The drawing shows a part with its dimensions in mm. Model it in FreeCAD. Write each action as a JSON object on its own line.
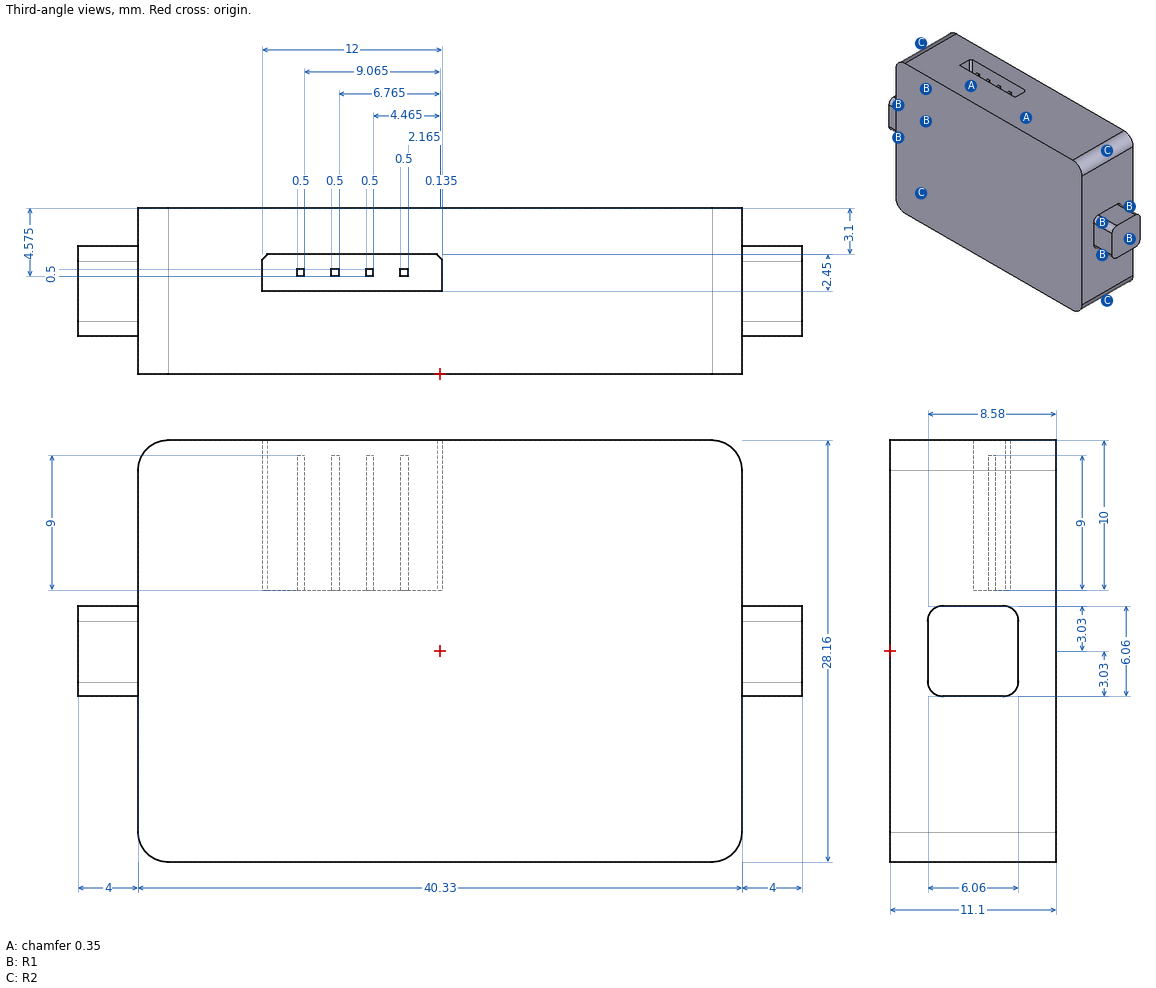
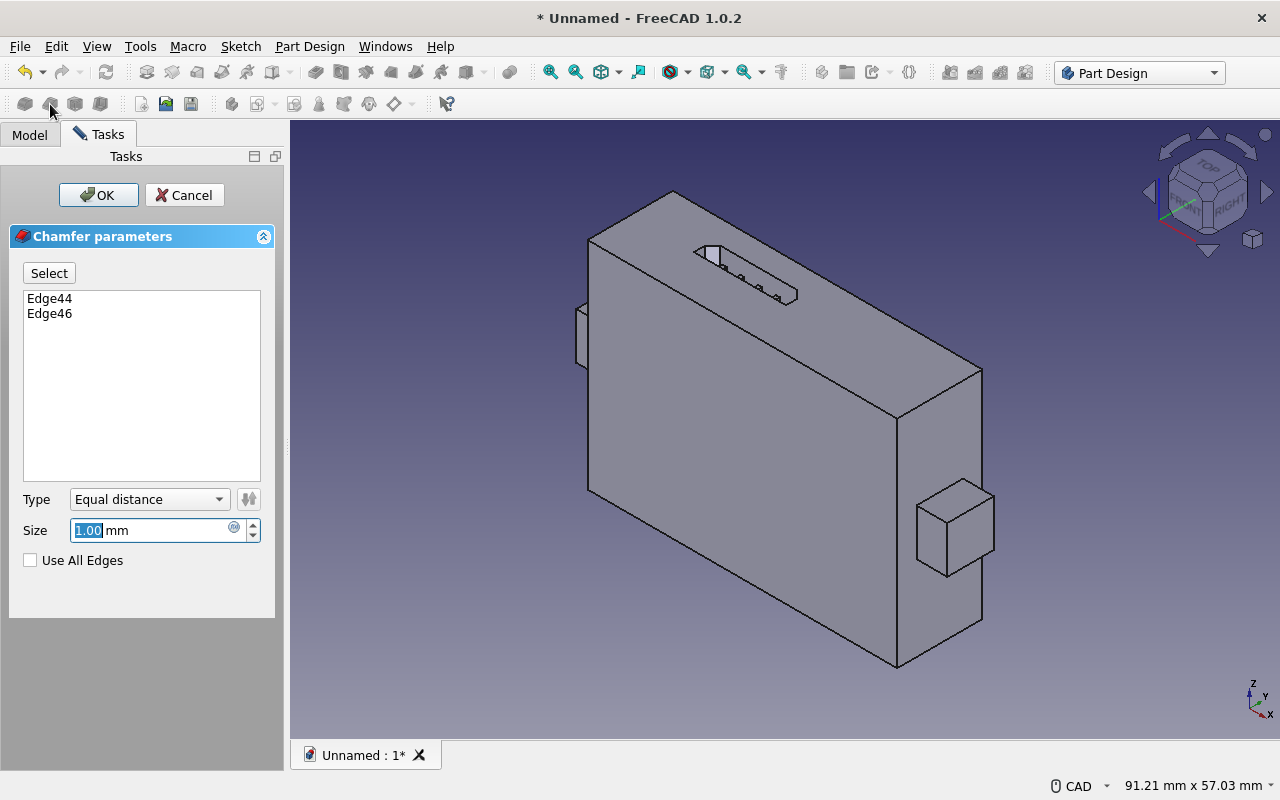
{"action": "type", "text": "0.35"}
{"action": "key", "text": "Tab"}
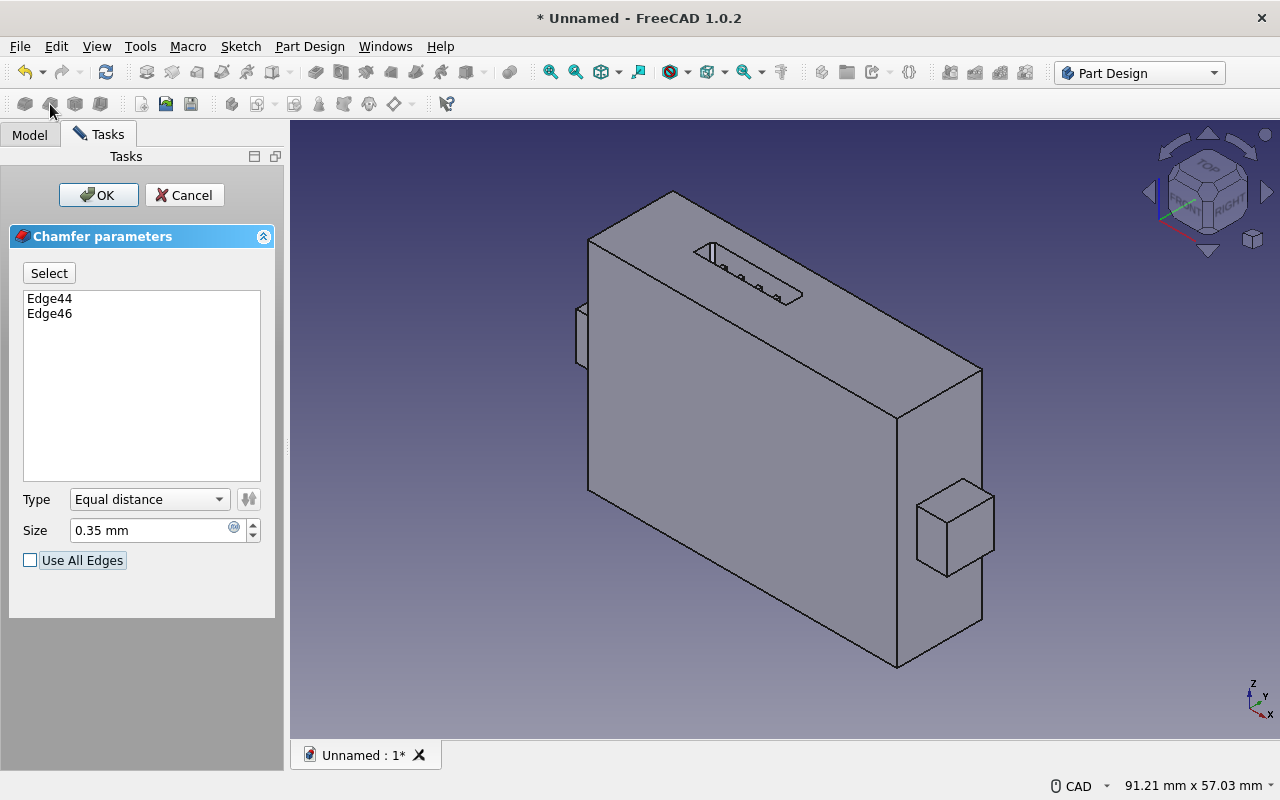
{"action": "left_click", "coordinate": [99, 195]}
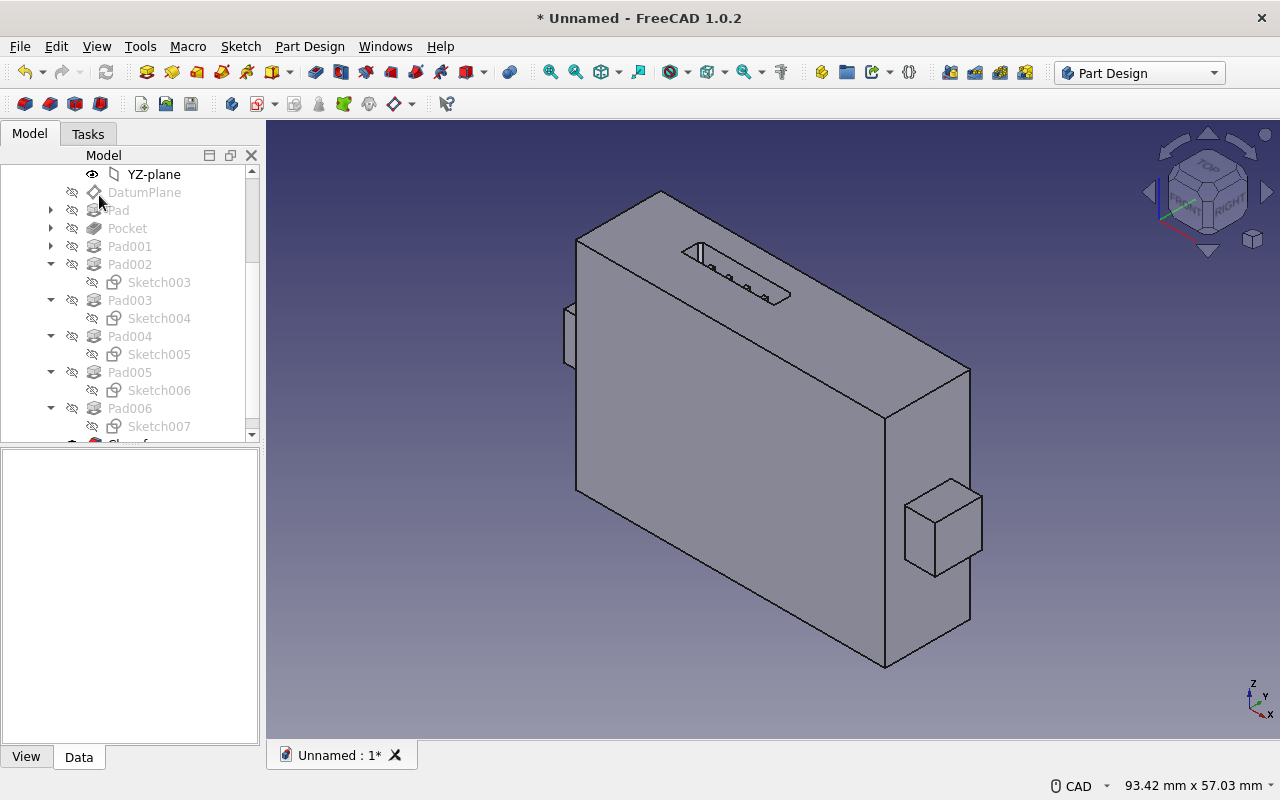
{"action": "left_click", "coordinate": [568, 310]}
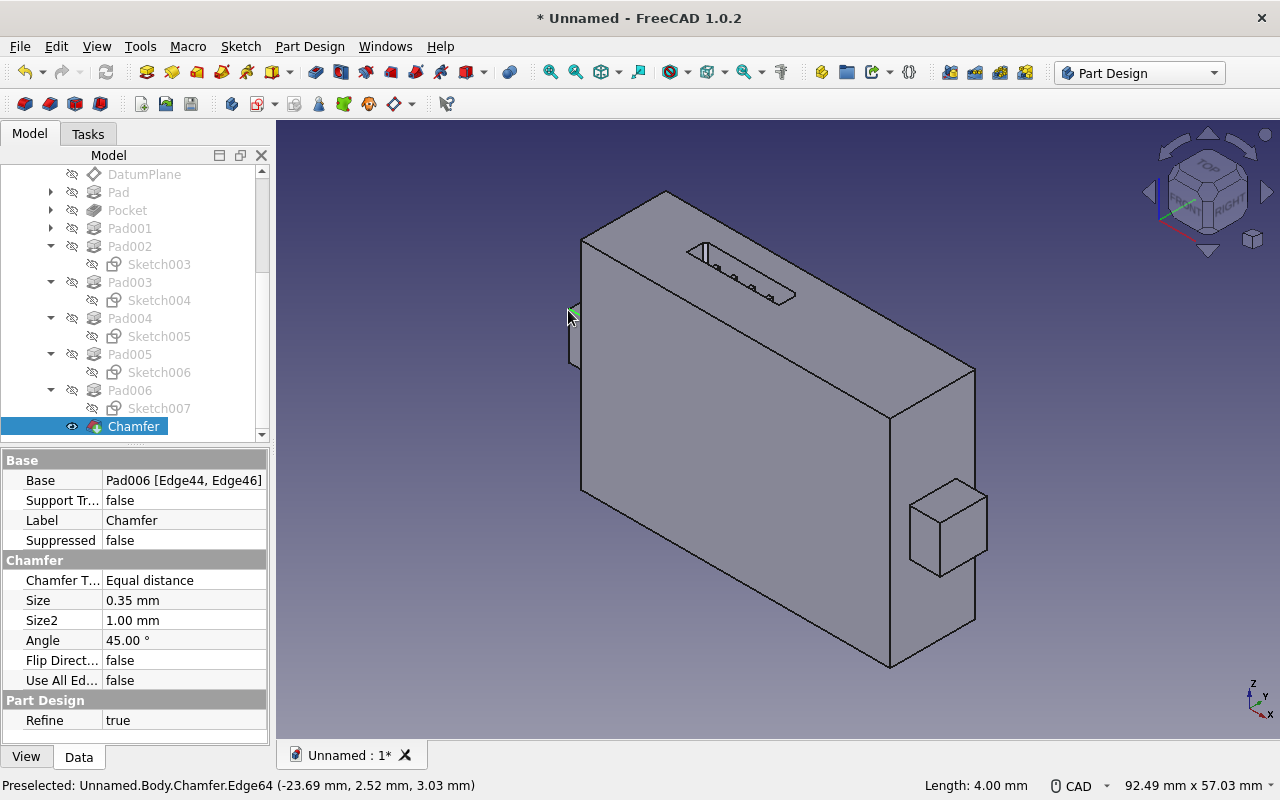
{"action": "left_click", "coordinate": [925, 513], "text": "ctrl"}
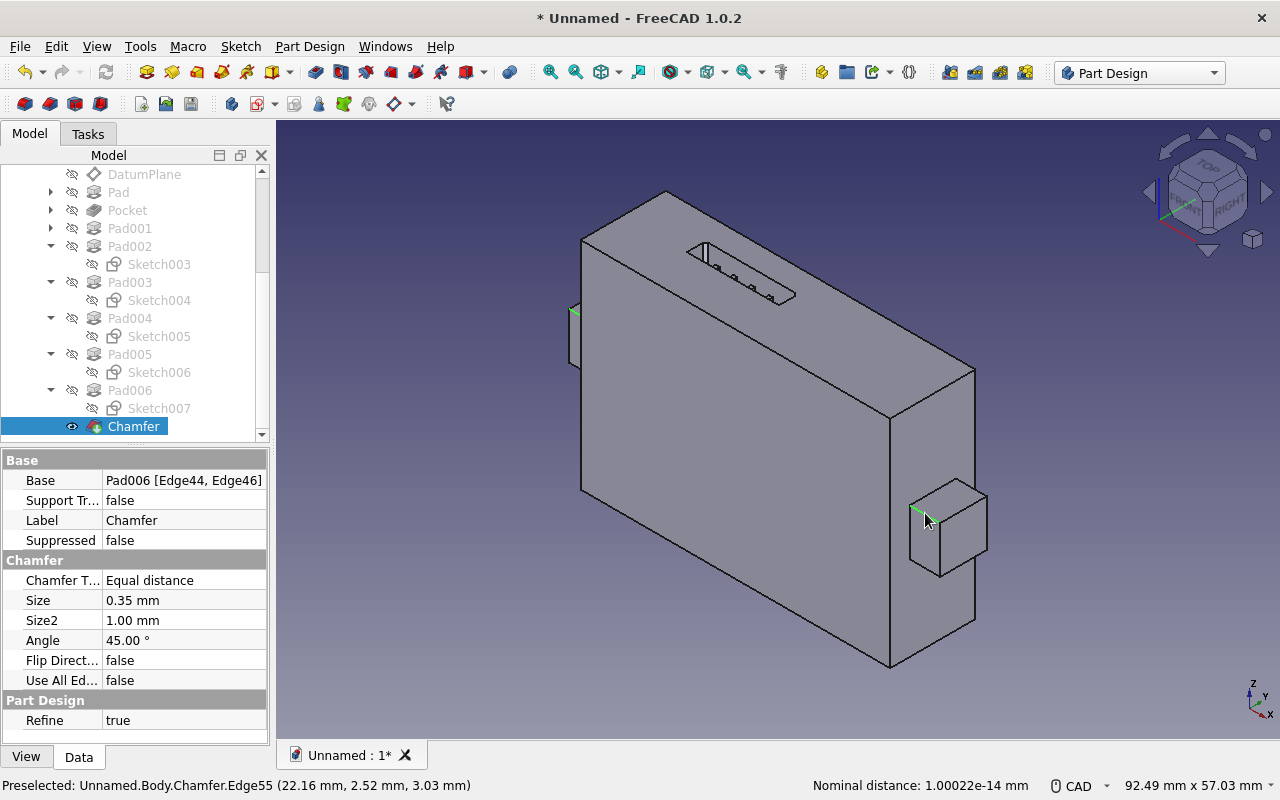
{"action": "key", "text": "2"}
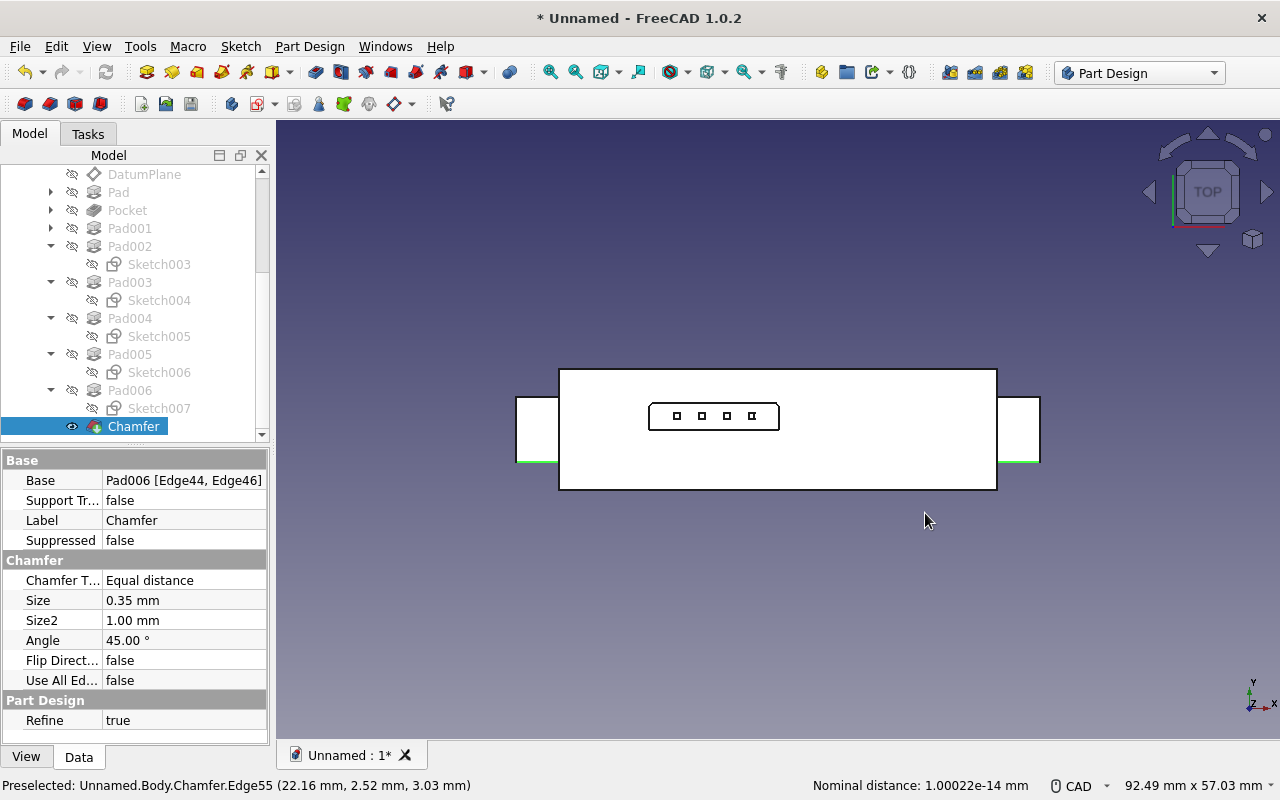
{"action": "left_click", "coordinate": [537, 396], "text": "ctrl"}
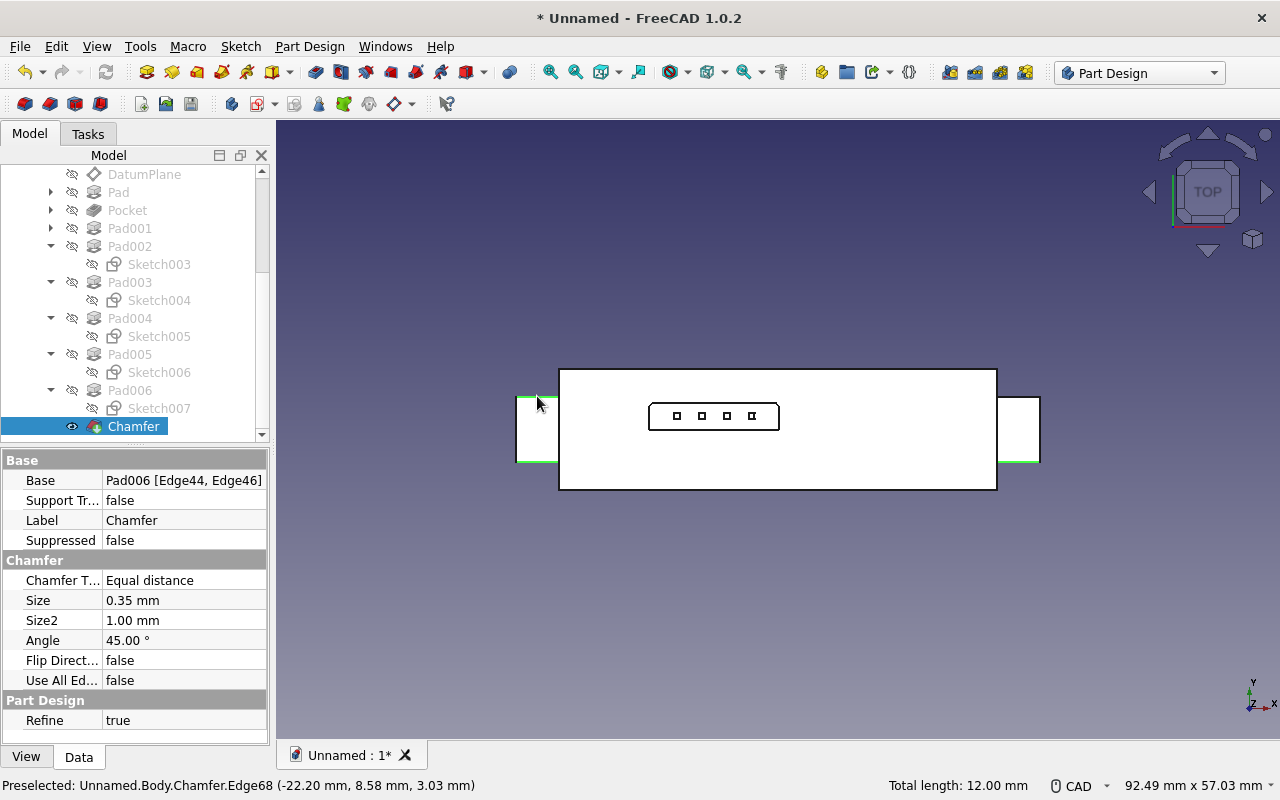
{"action": "left_click", "coordinate": [1019, 396], "text": "ctrl"}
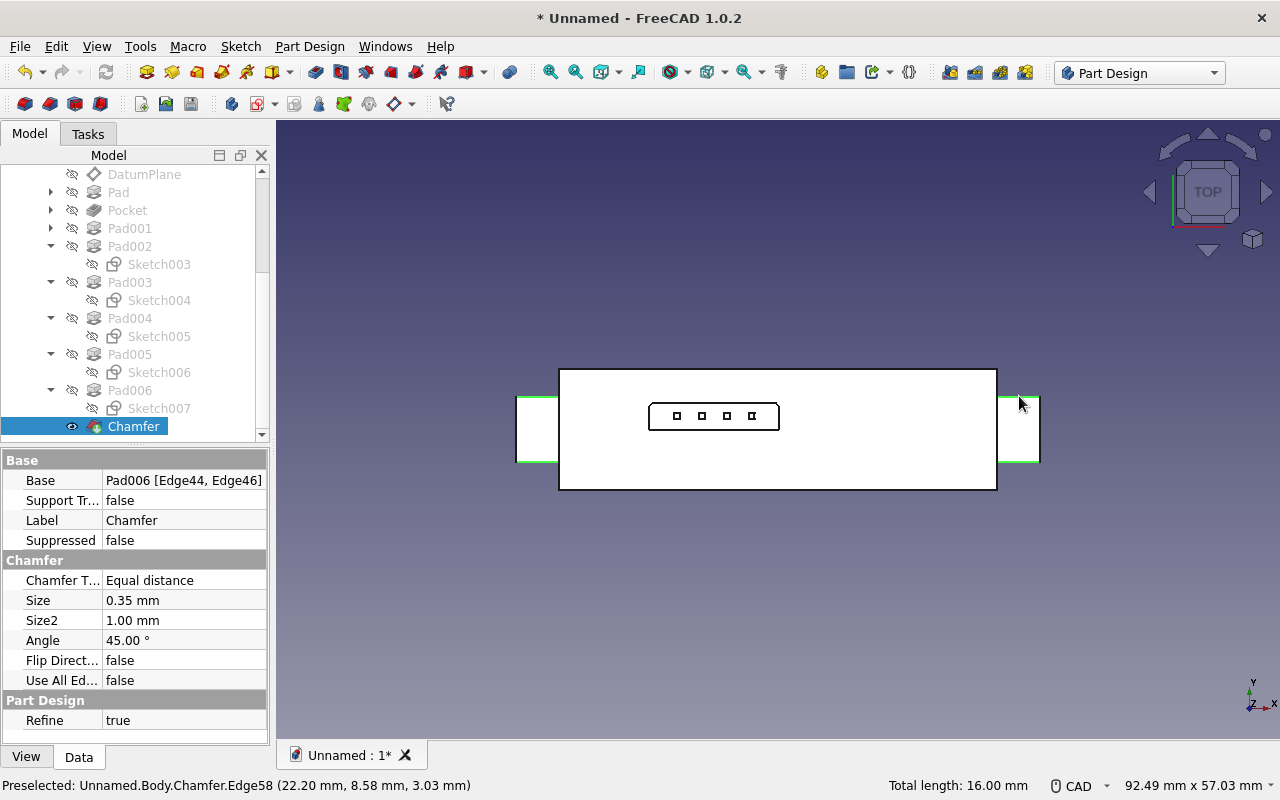
{"action": "key", "text": "0"}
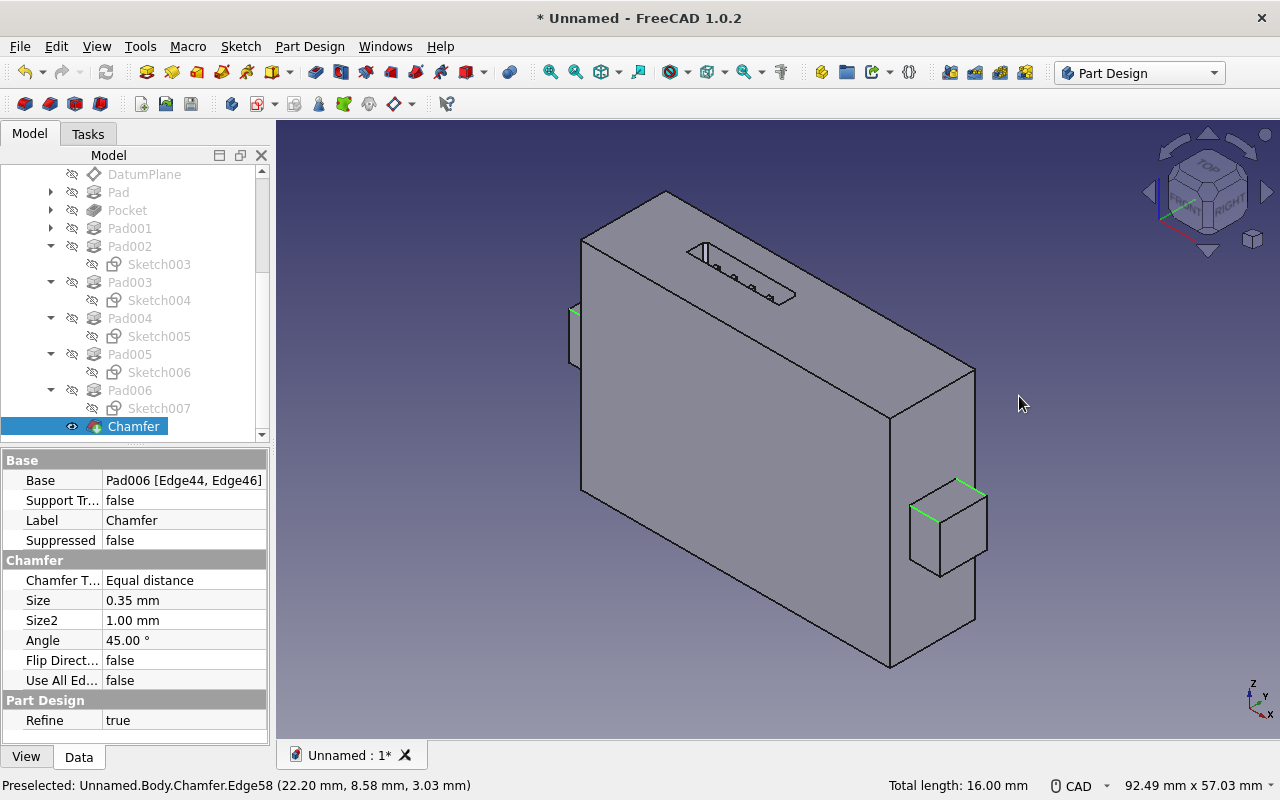
{"action": "key", "text": "1"}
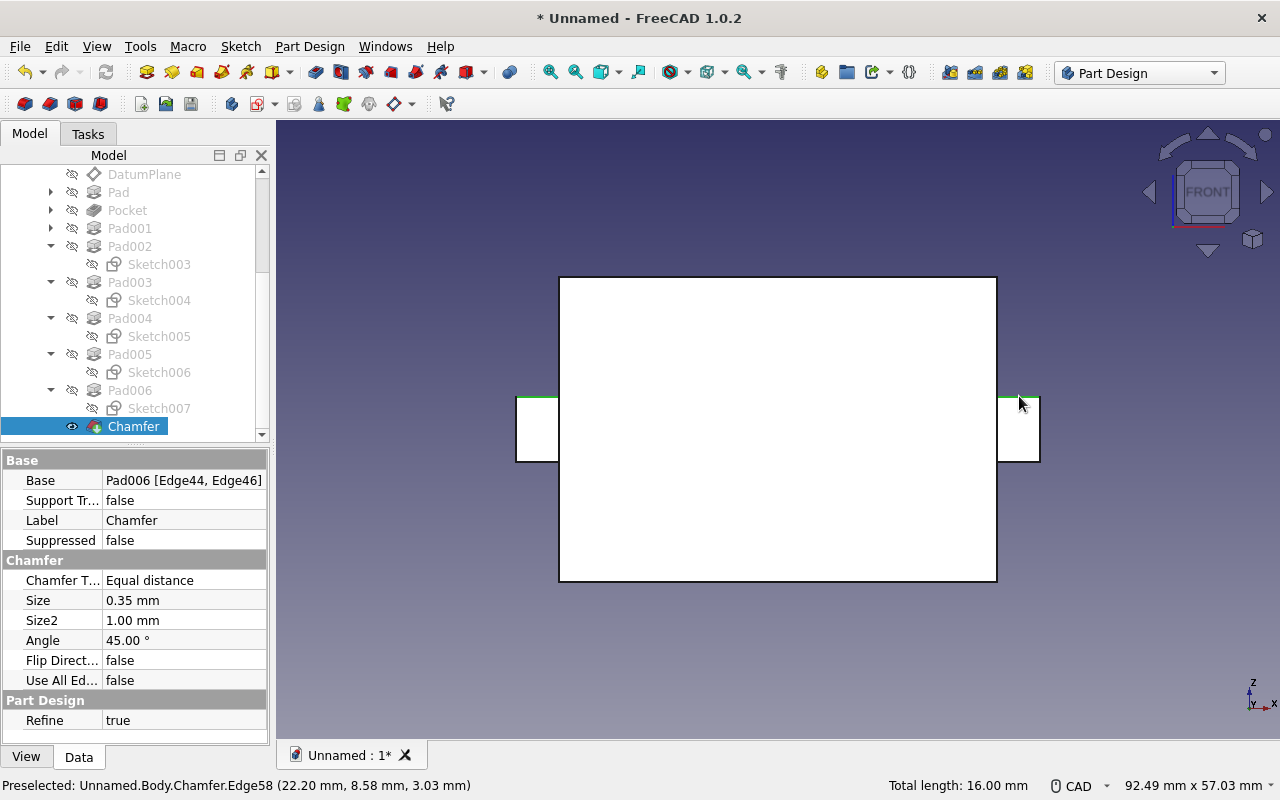
{"action": "key", "text": "3"}